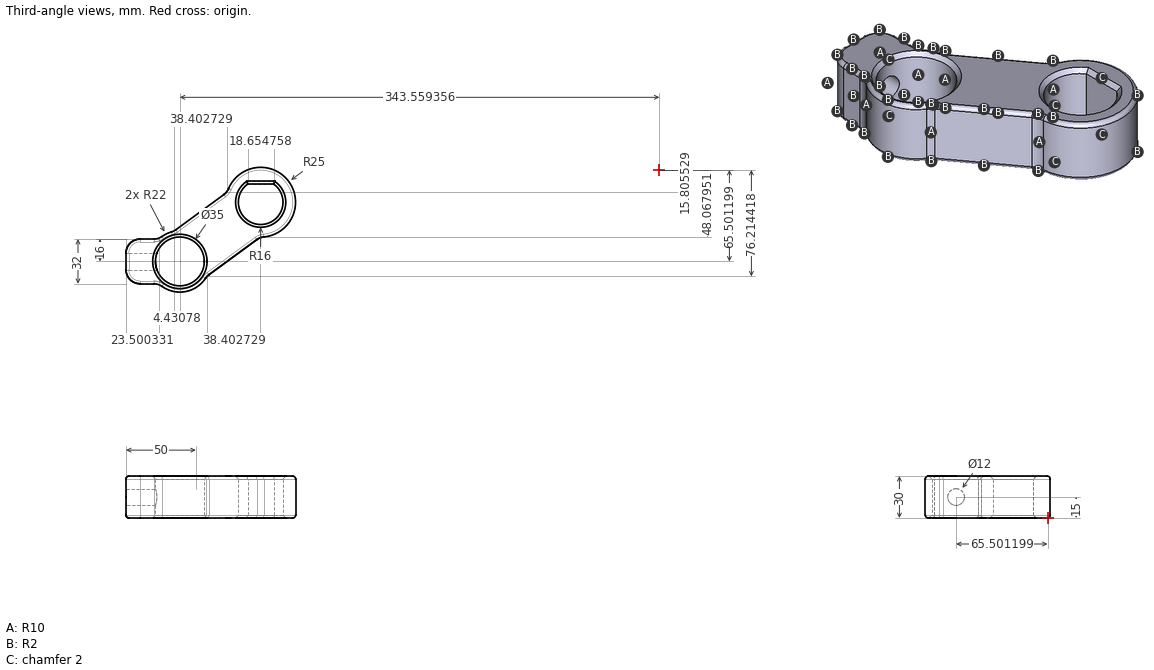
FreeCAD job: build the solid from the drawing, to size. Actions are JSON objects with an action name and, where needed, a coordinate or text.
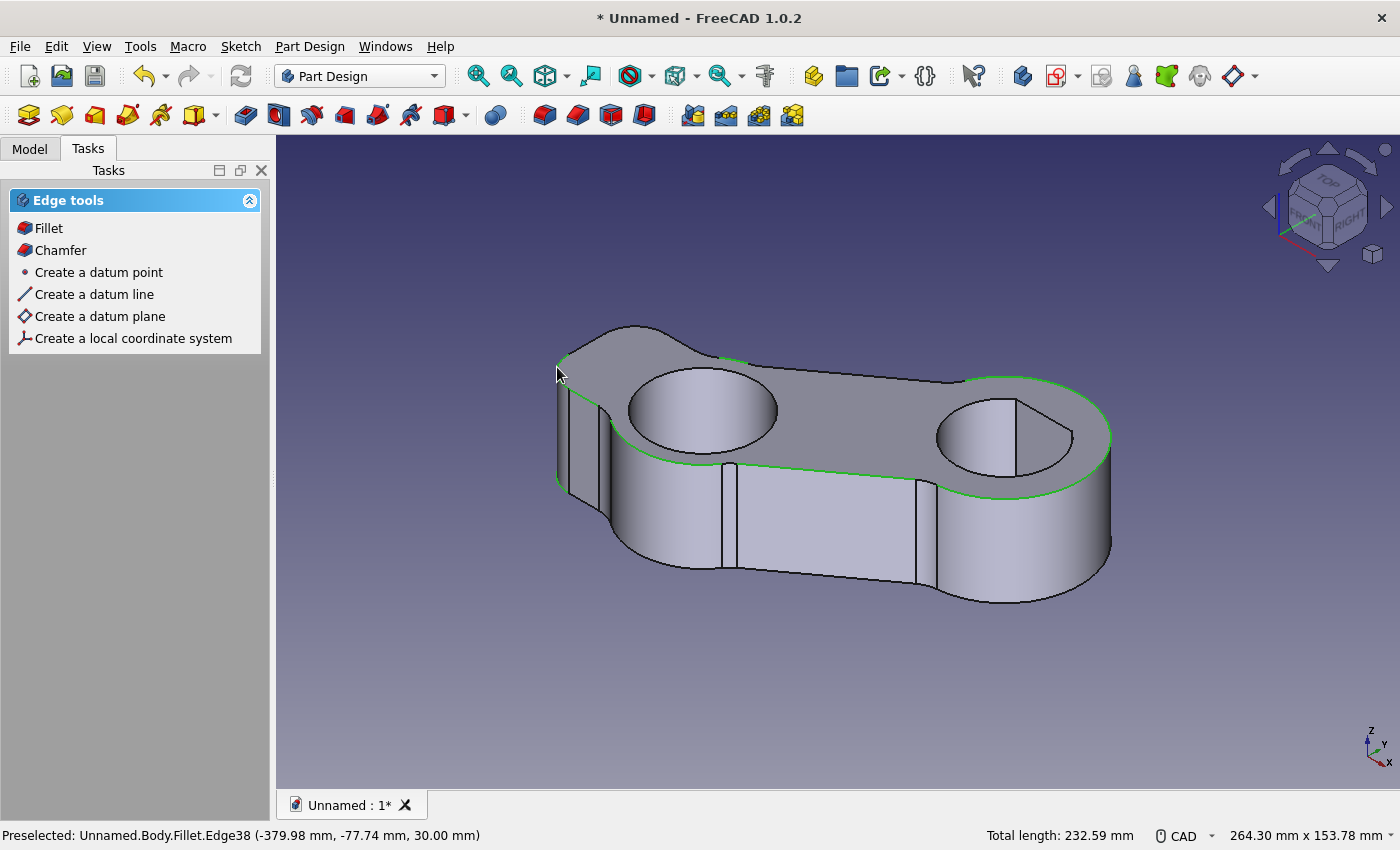
{"action": "left_click", "coordinate": [750, 363], "text": "ctrl"}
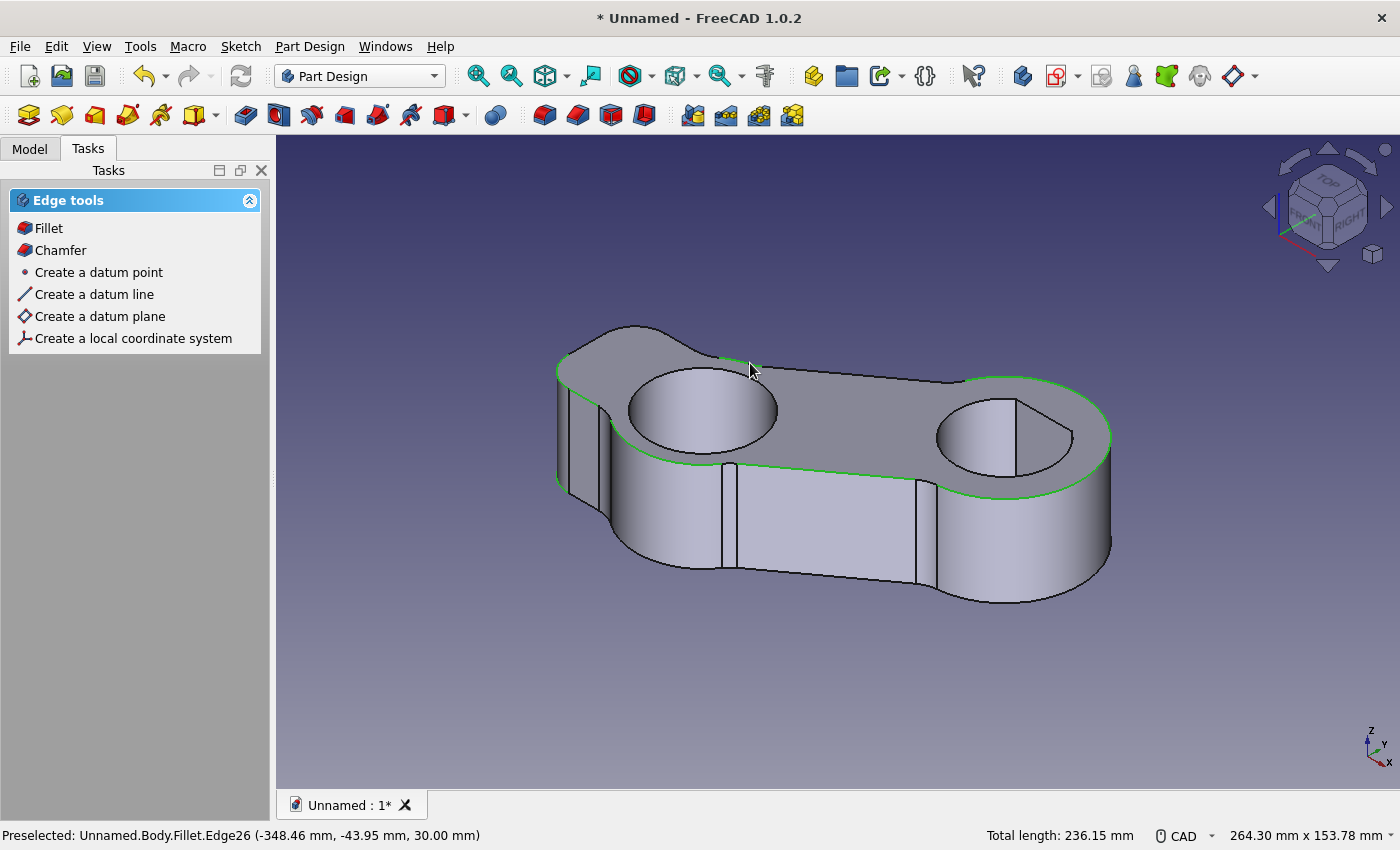
{"action": "left_click", "coordinate": [729, 462], "text": "ctrl"}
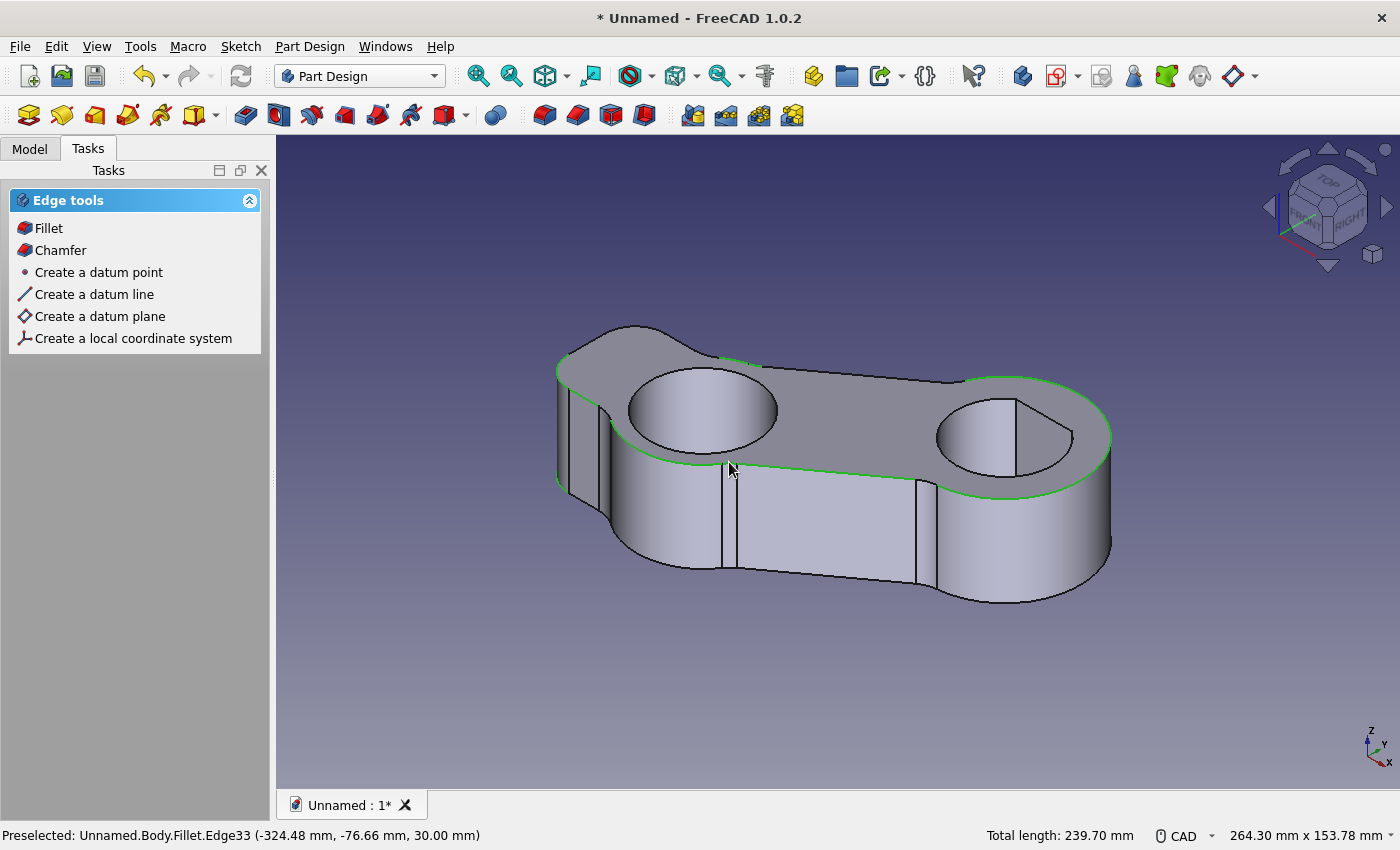
{"action": "left_click", "coordinate": [607, 411], "text": "ctrl"}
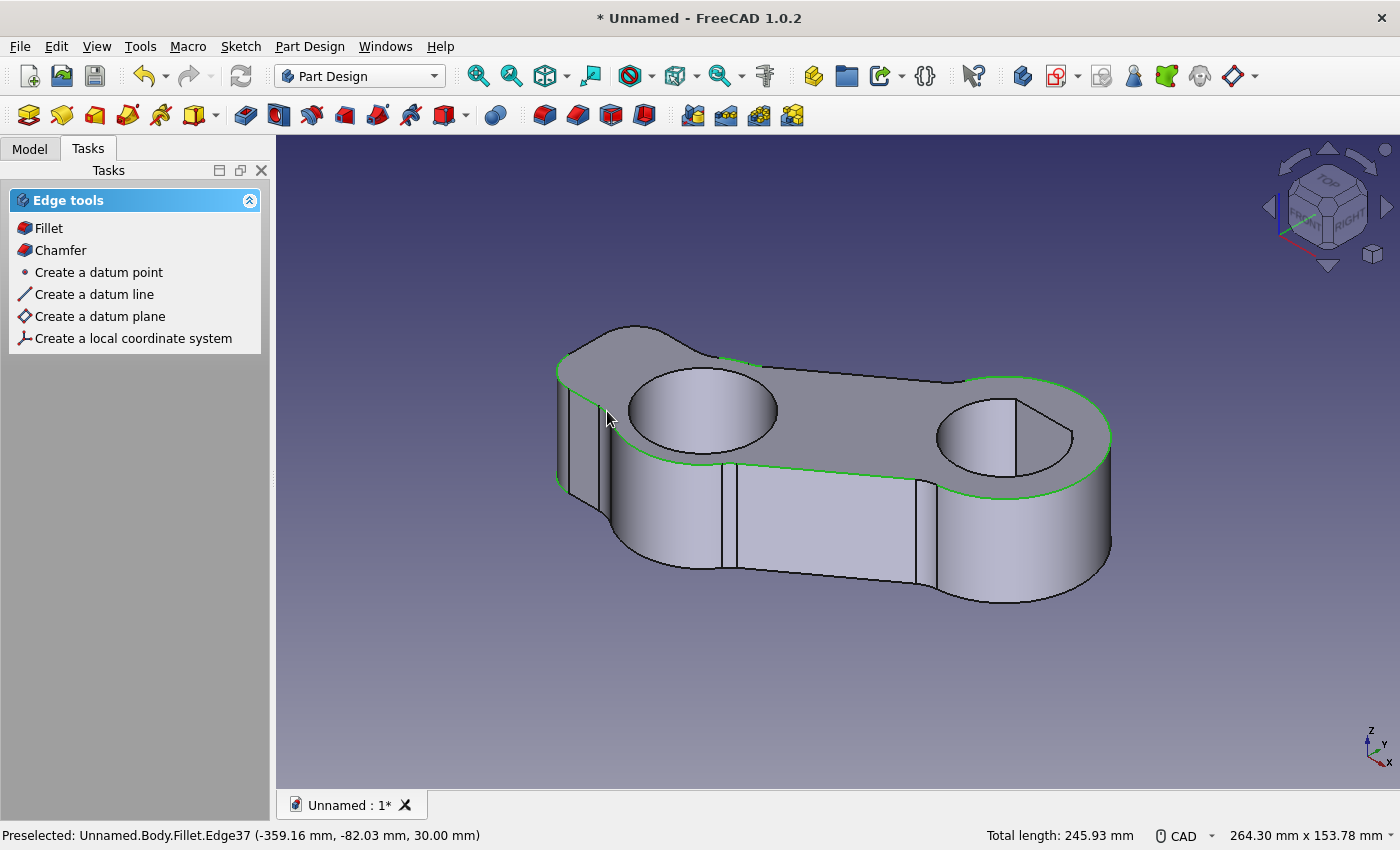
{"action": "left_click", "coordinate": [706, 354], "text": "ctrl"}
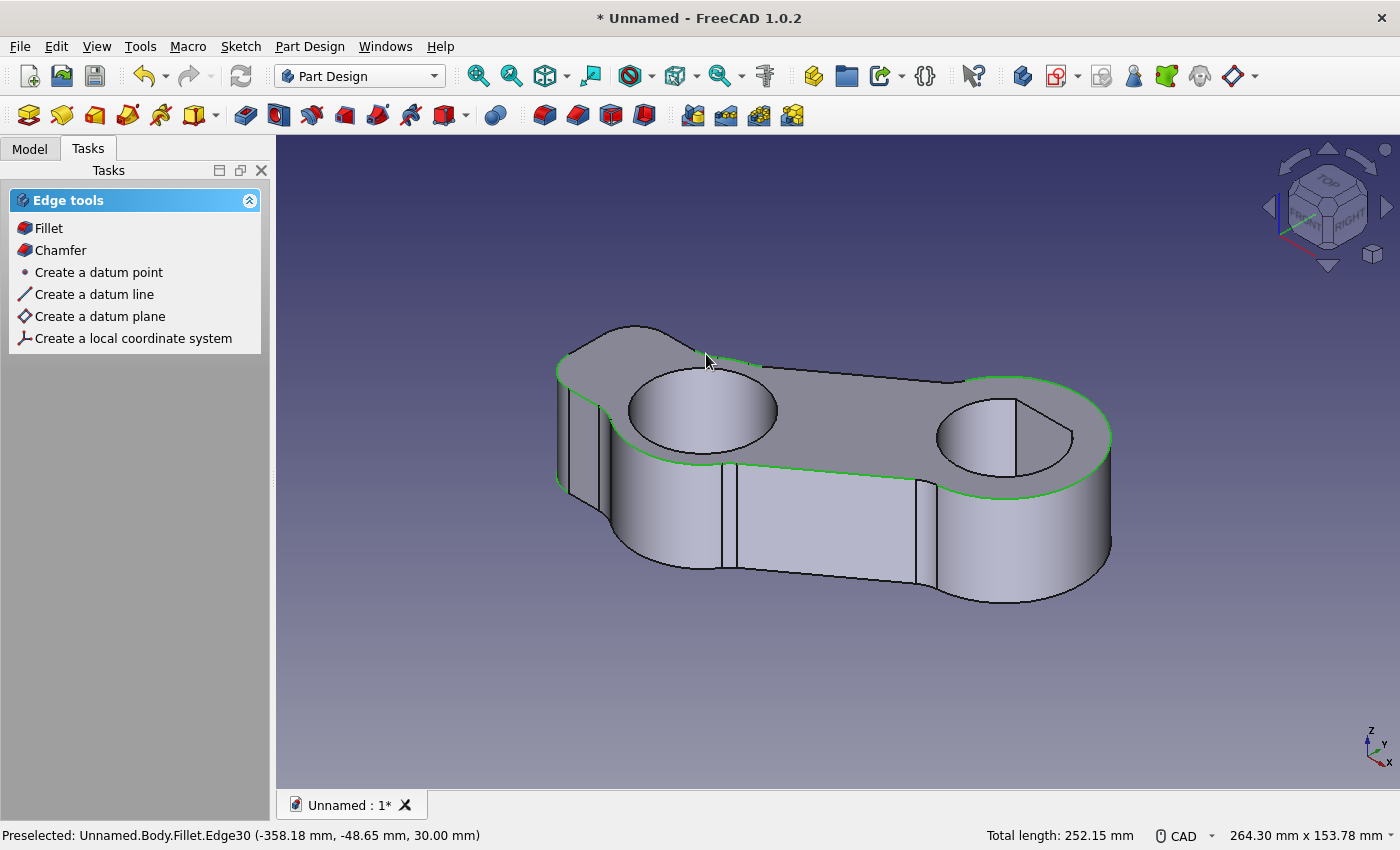
{"action": "left_click", "coordinate": [927, 480], "text": "ctrl"}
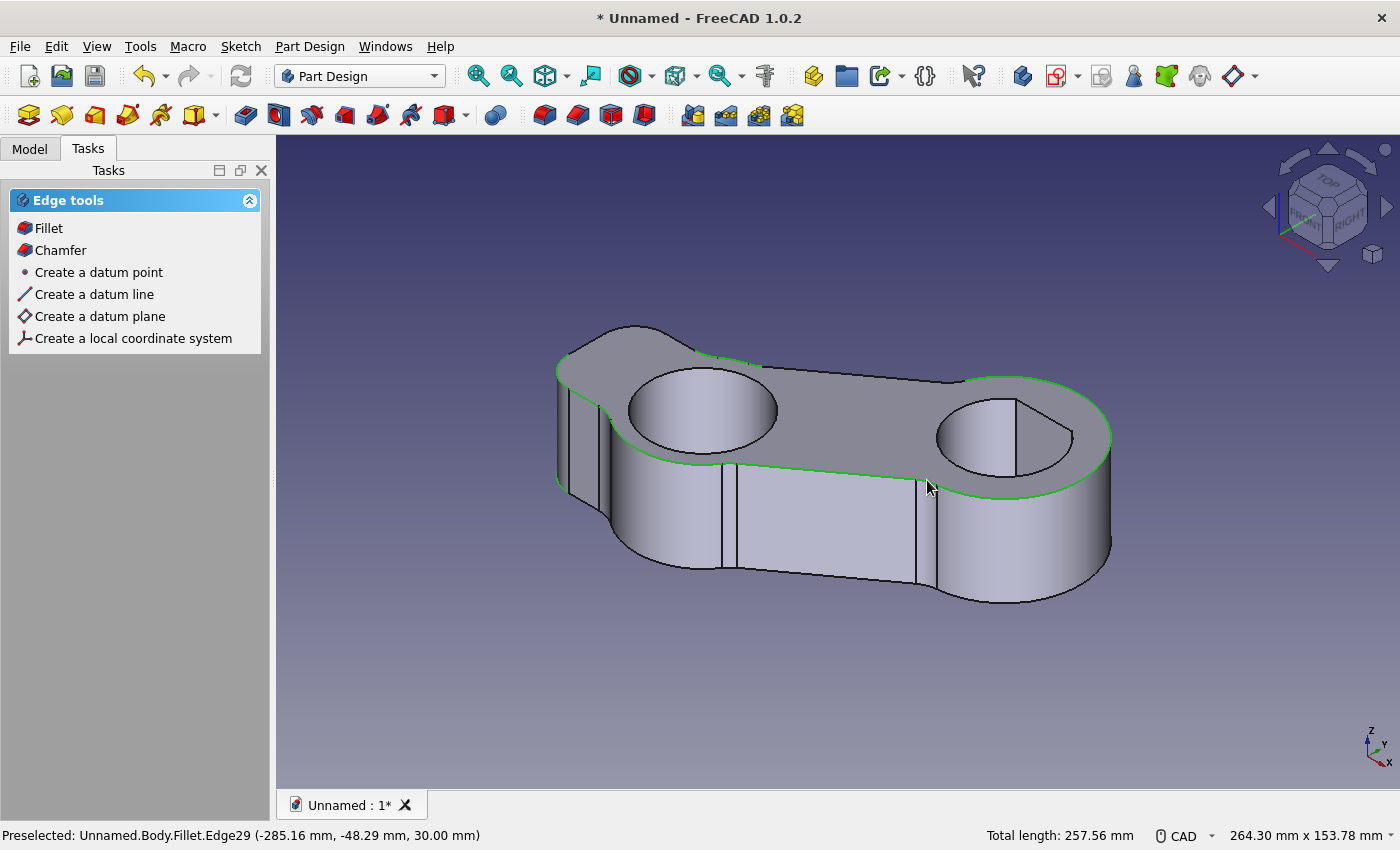
{"action": "key", "text": "2"}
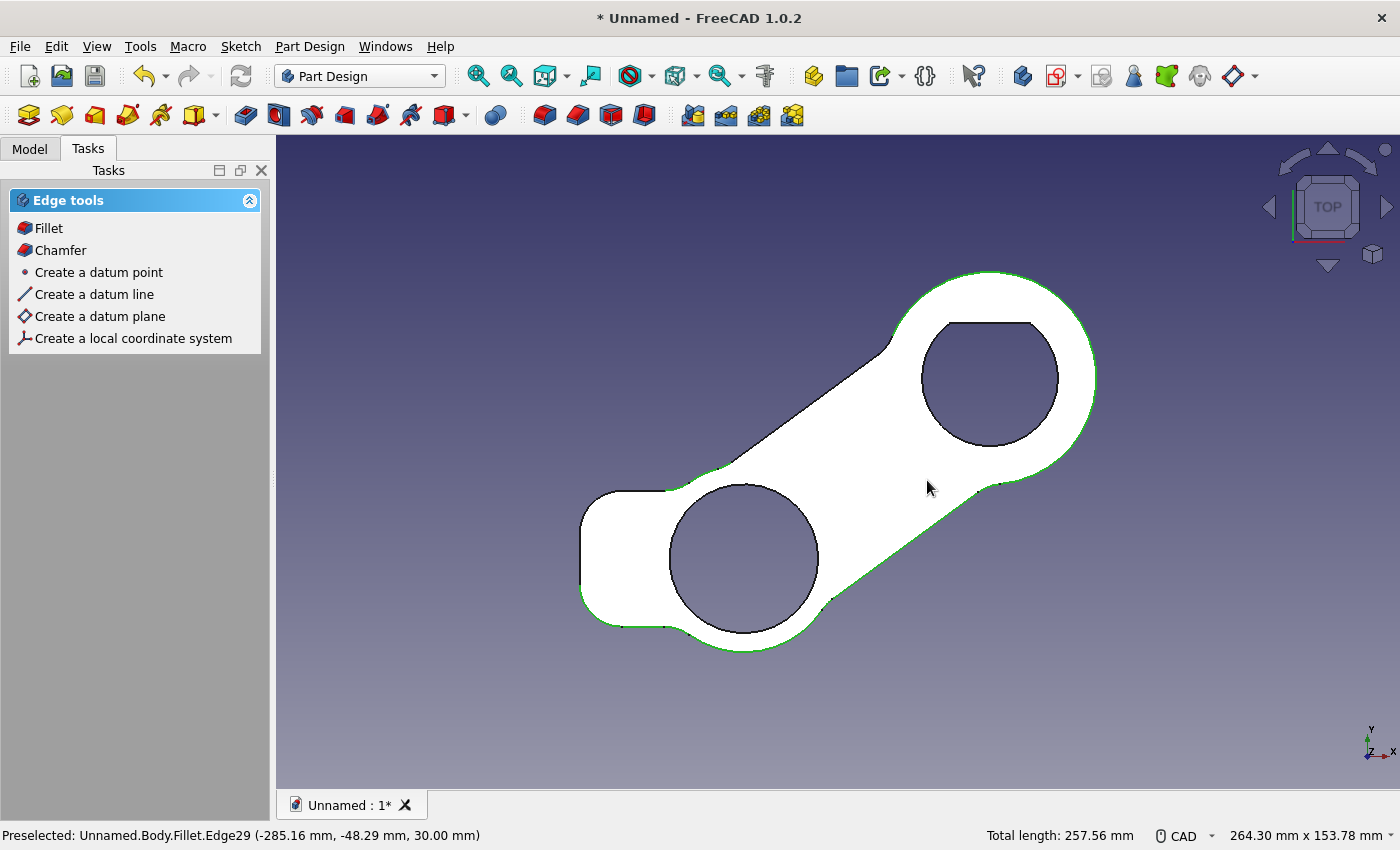
{"action": "left_click", "coordinate": [805, 408], "text": "ctrl"}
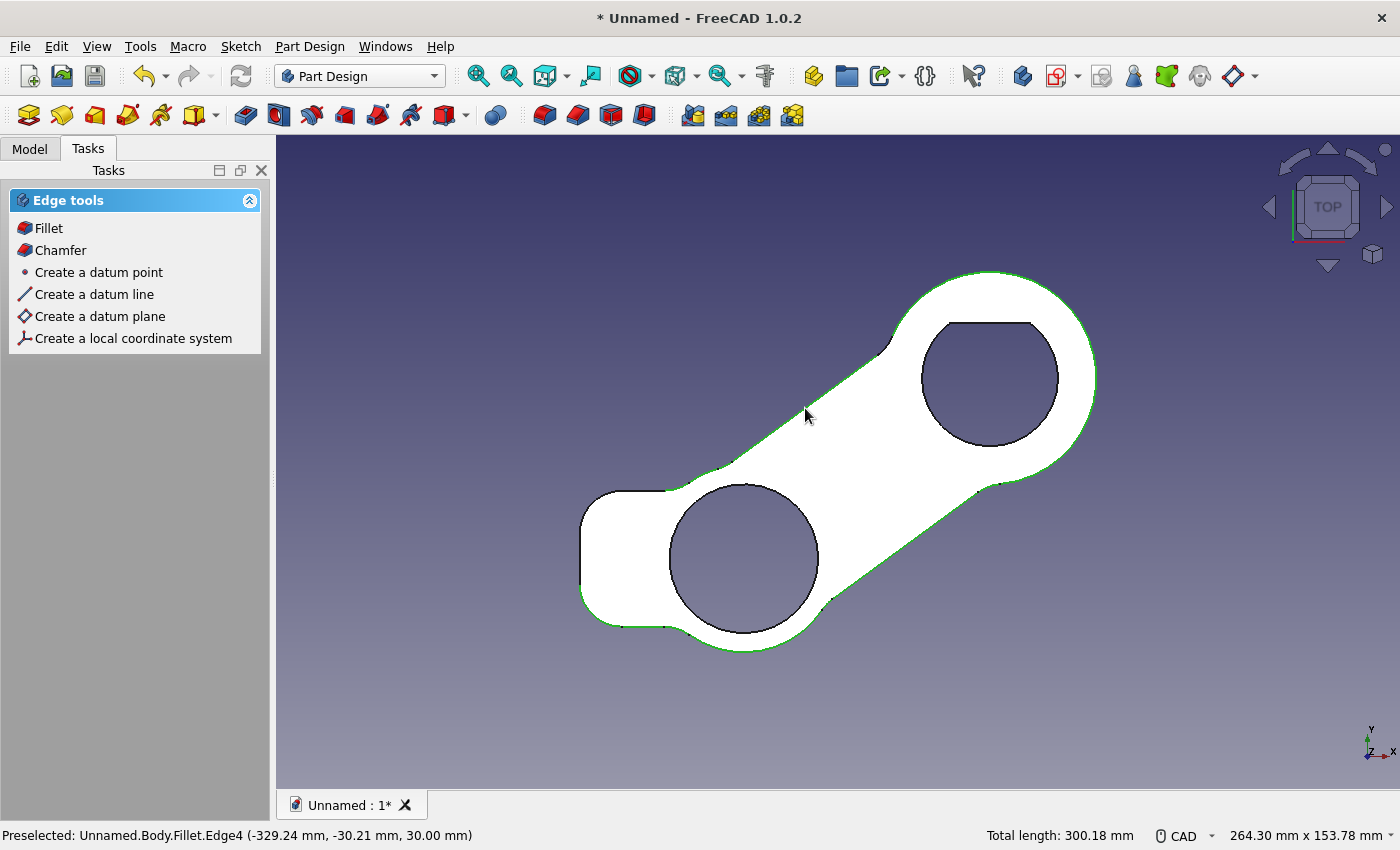
{"action": "left_click", "coordinate": [580, 558], "text": "ctrl"}